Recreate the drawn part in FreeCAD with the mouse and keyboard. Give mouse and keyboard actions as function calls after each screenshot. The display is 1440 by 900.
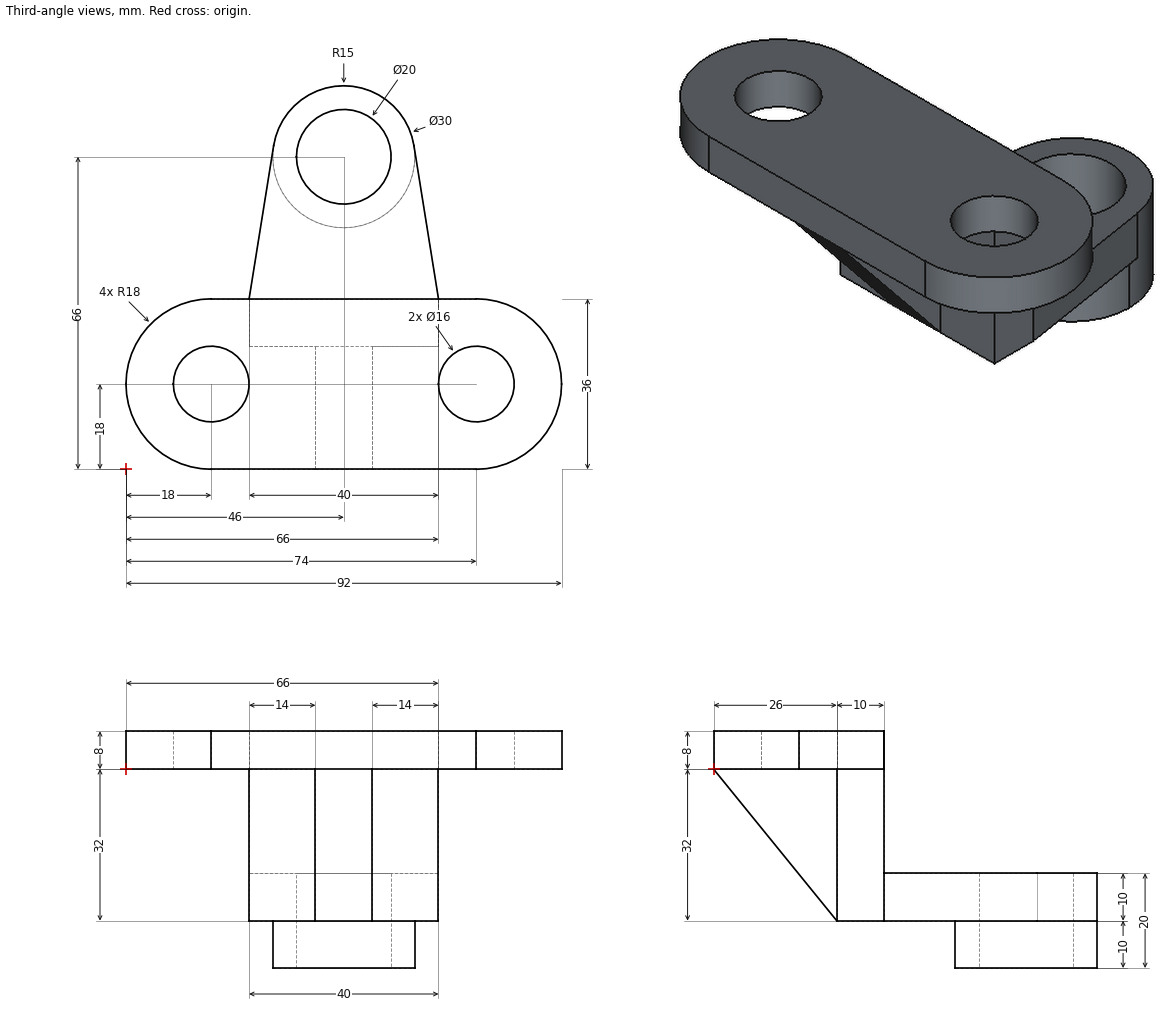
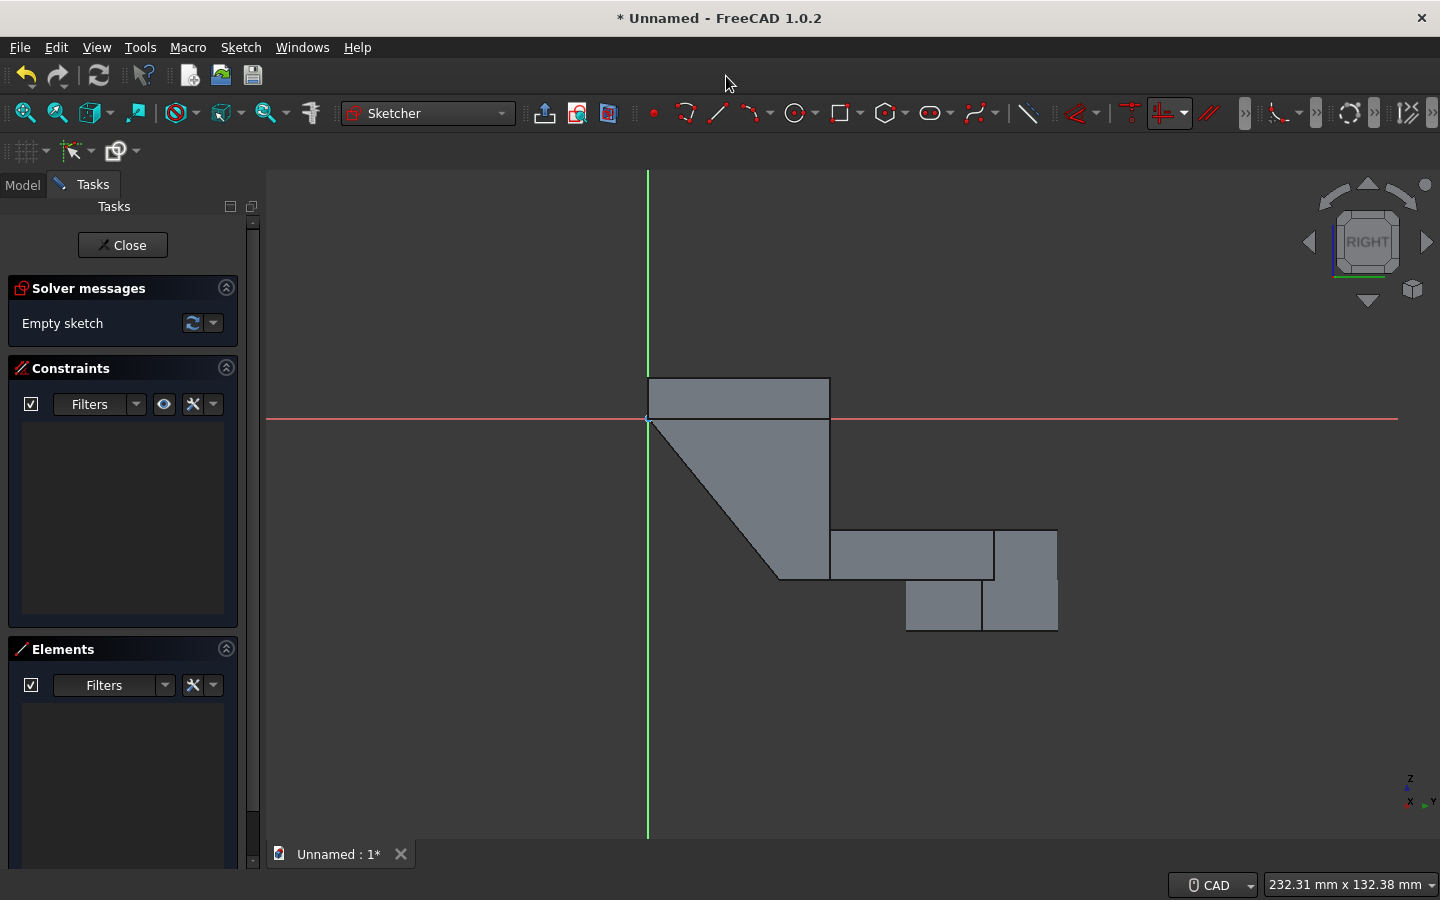
click(610, 114)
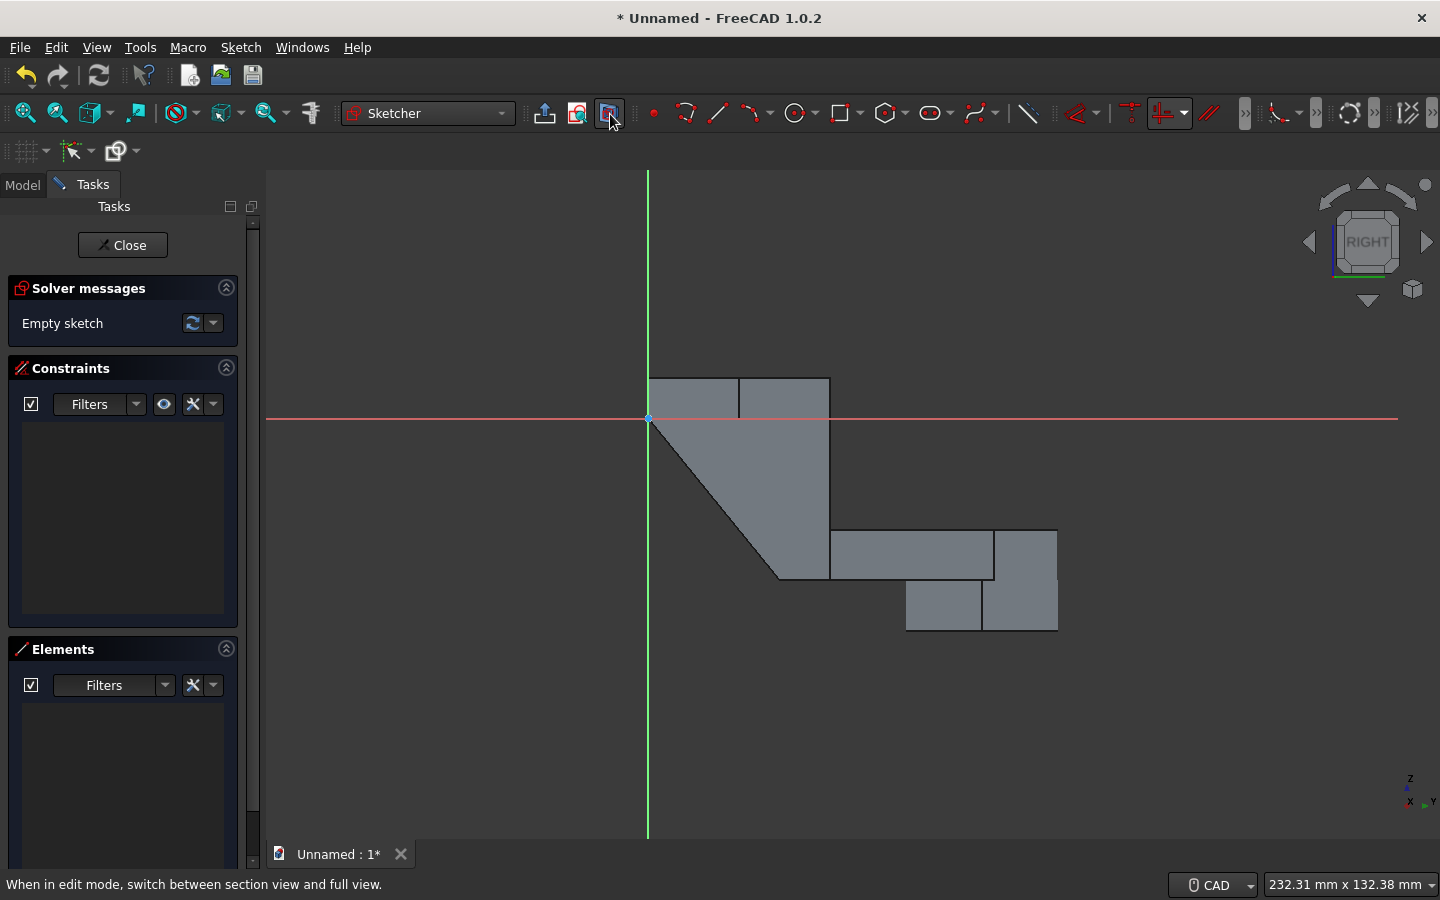
scroll(673, 497, up, 5)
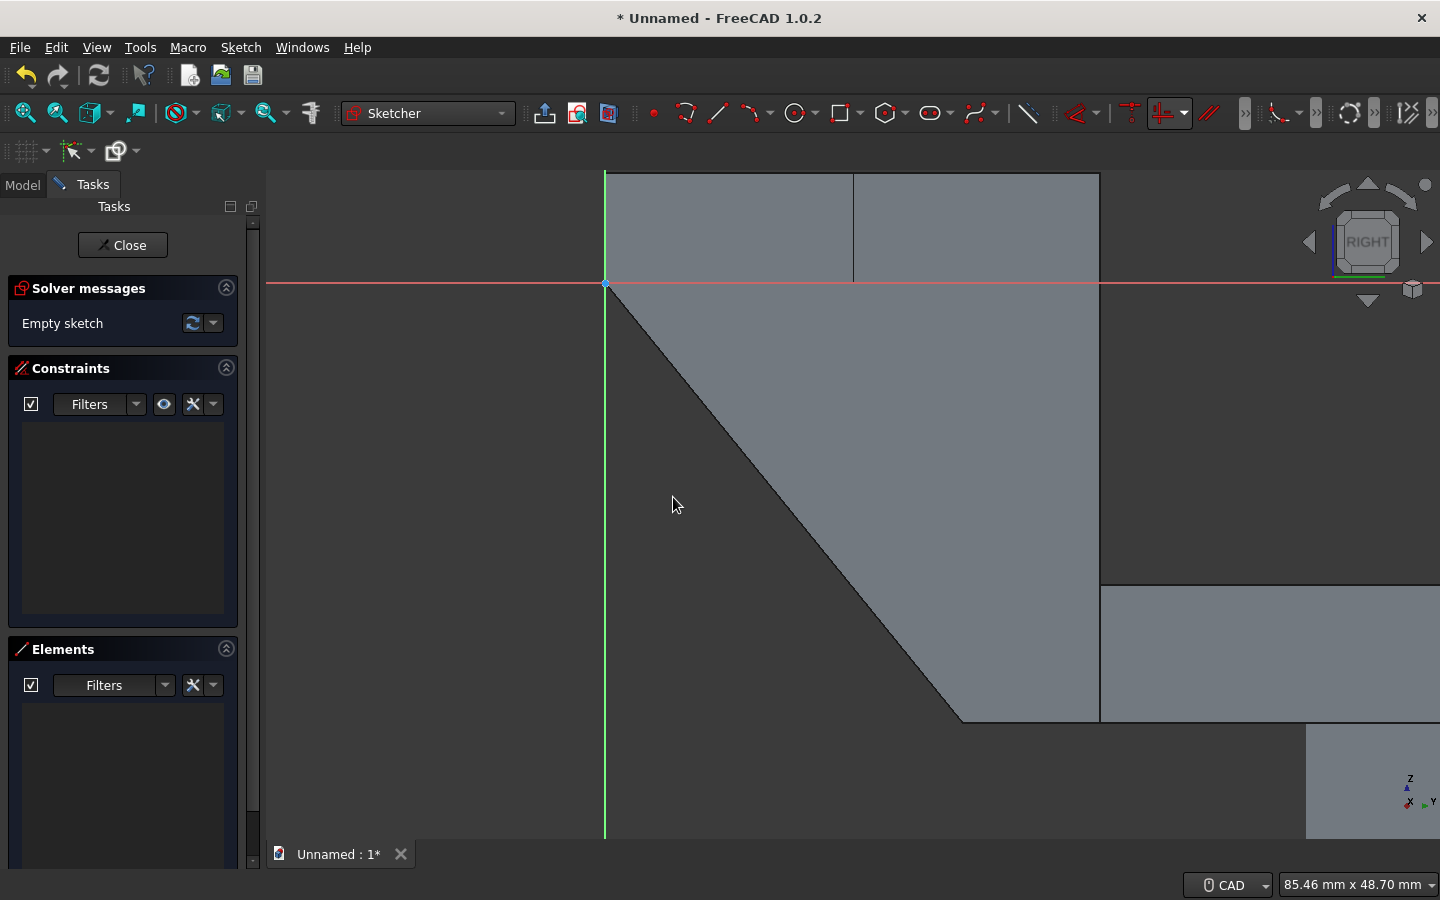
click(686, 114)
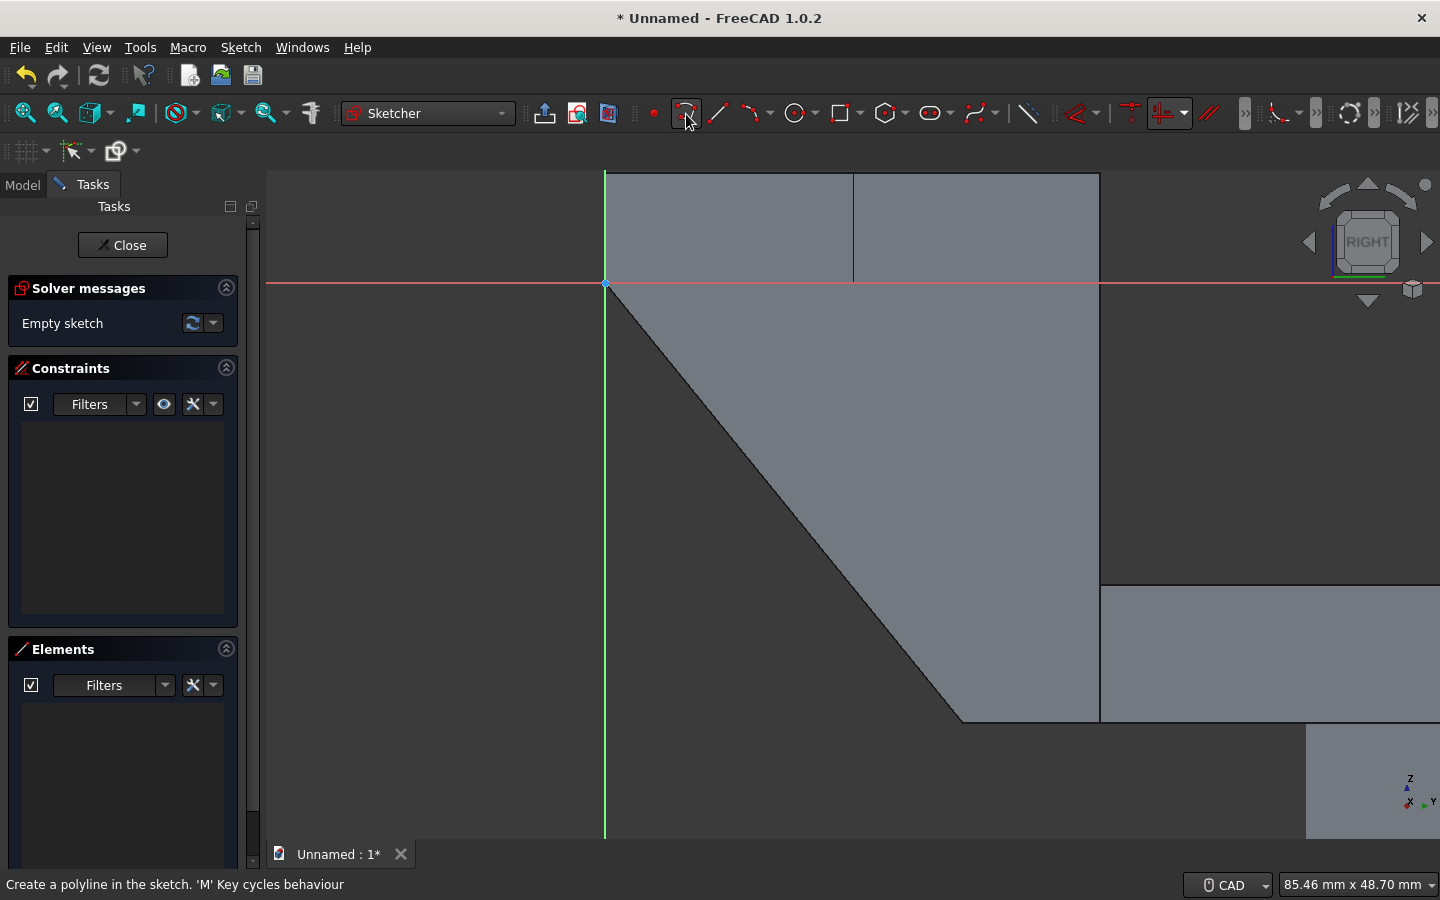
click(605, 283)
click(963, 723)
click(963, 292)
click(605, 283)
key(Escape)
key(Escape)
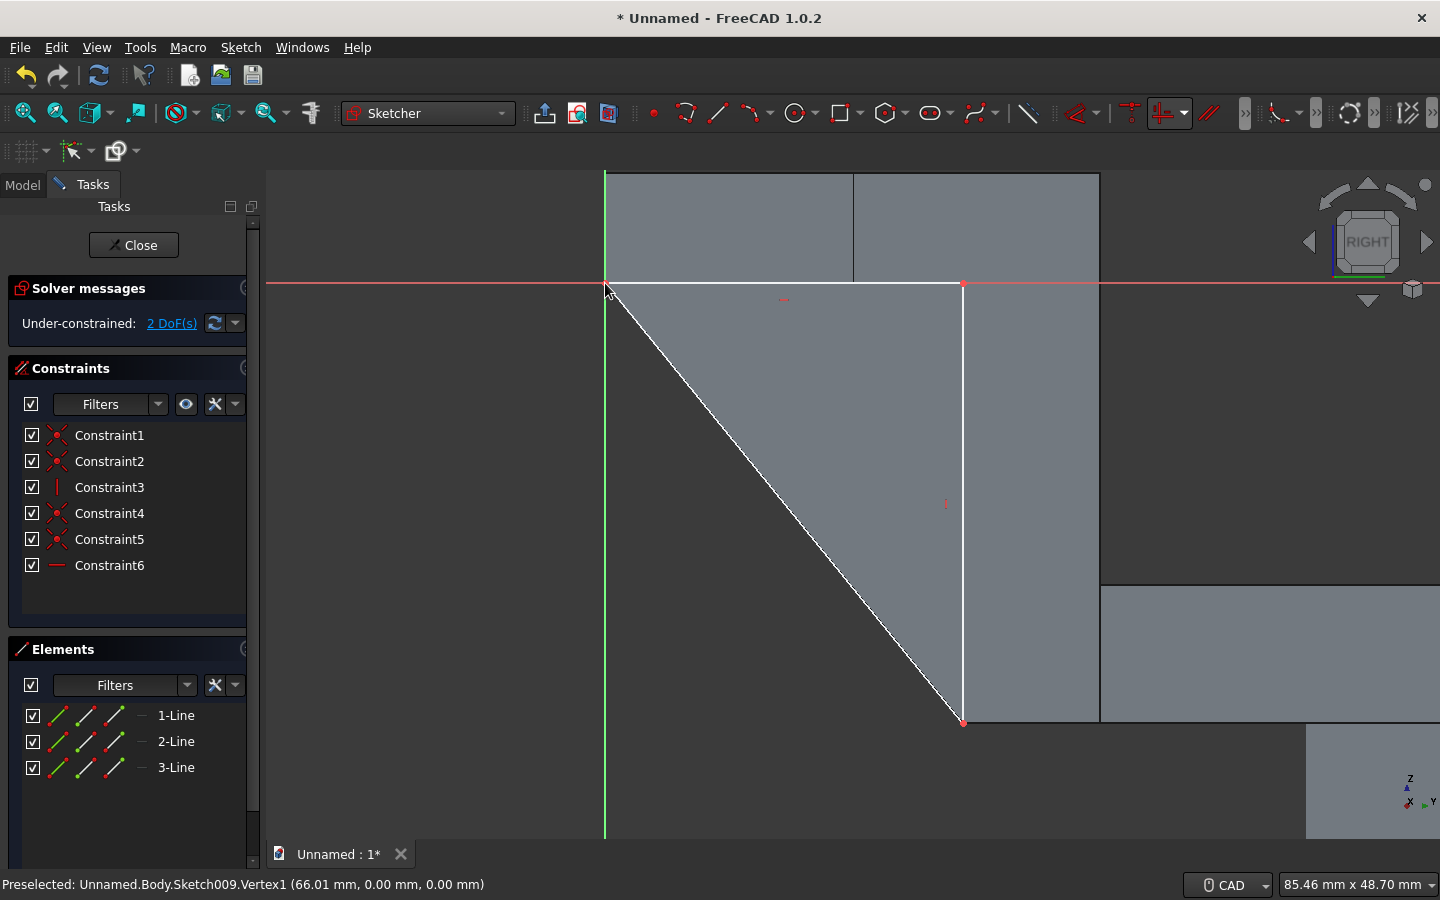
click(1076, 114)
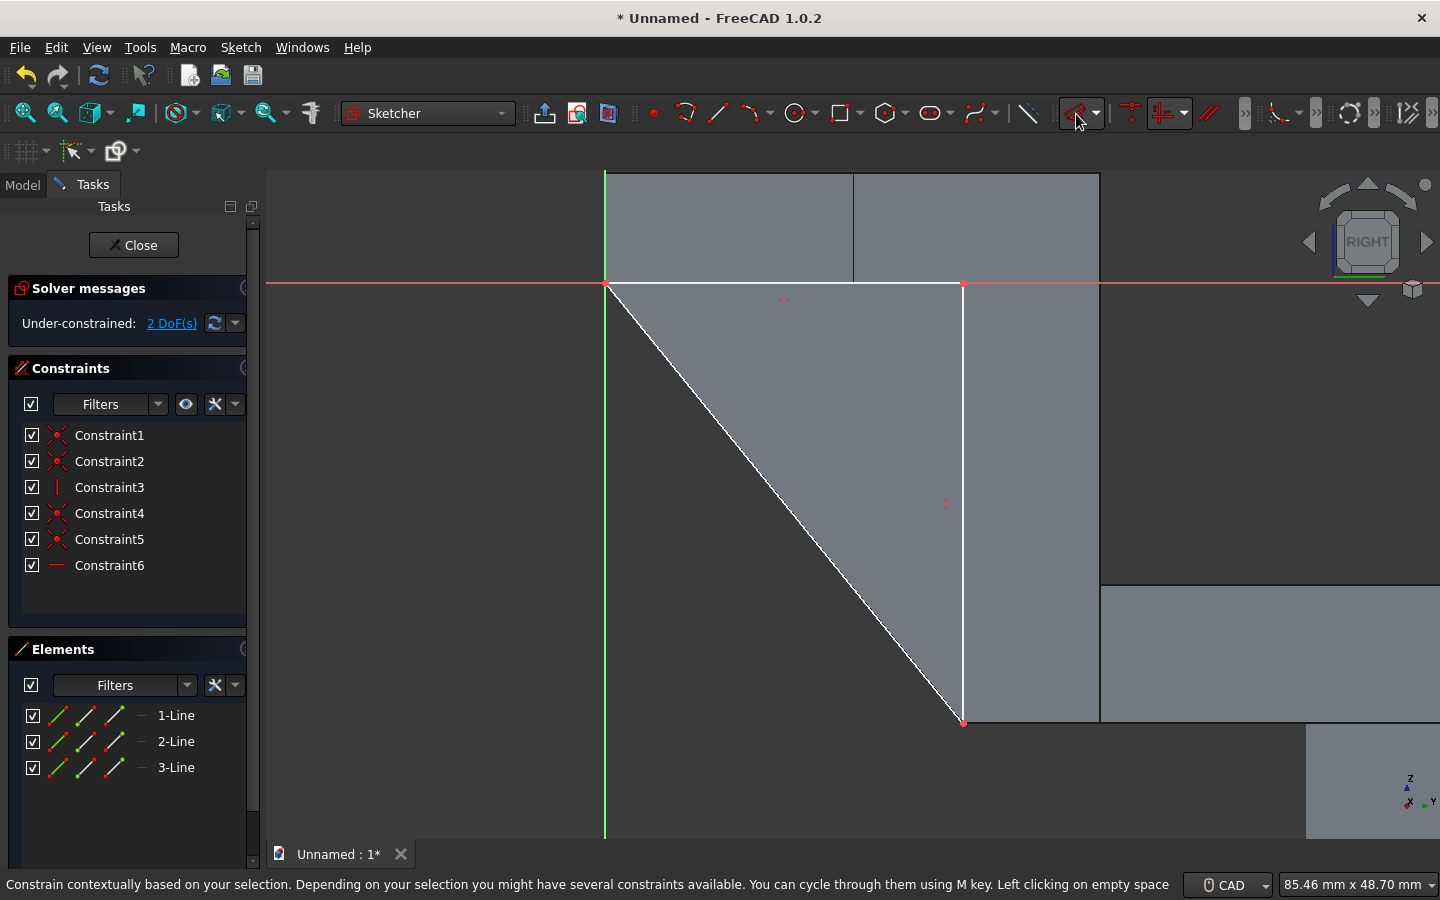
click(963, 592)
click(997, 504)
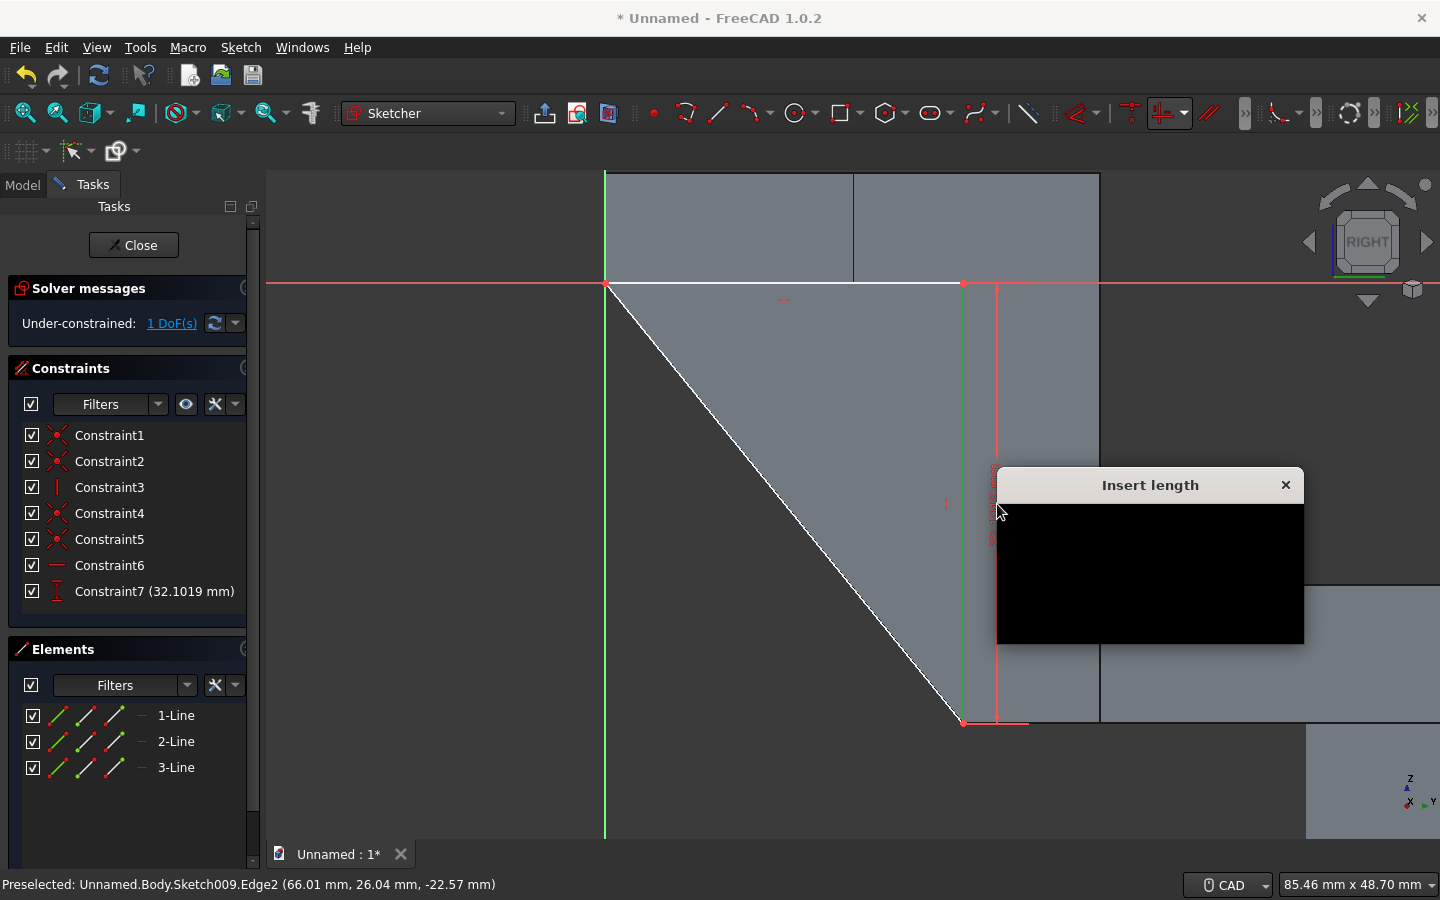
text(32)
key(Return)